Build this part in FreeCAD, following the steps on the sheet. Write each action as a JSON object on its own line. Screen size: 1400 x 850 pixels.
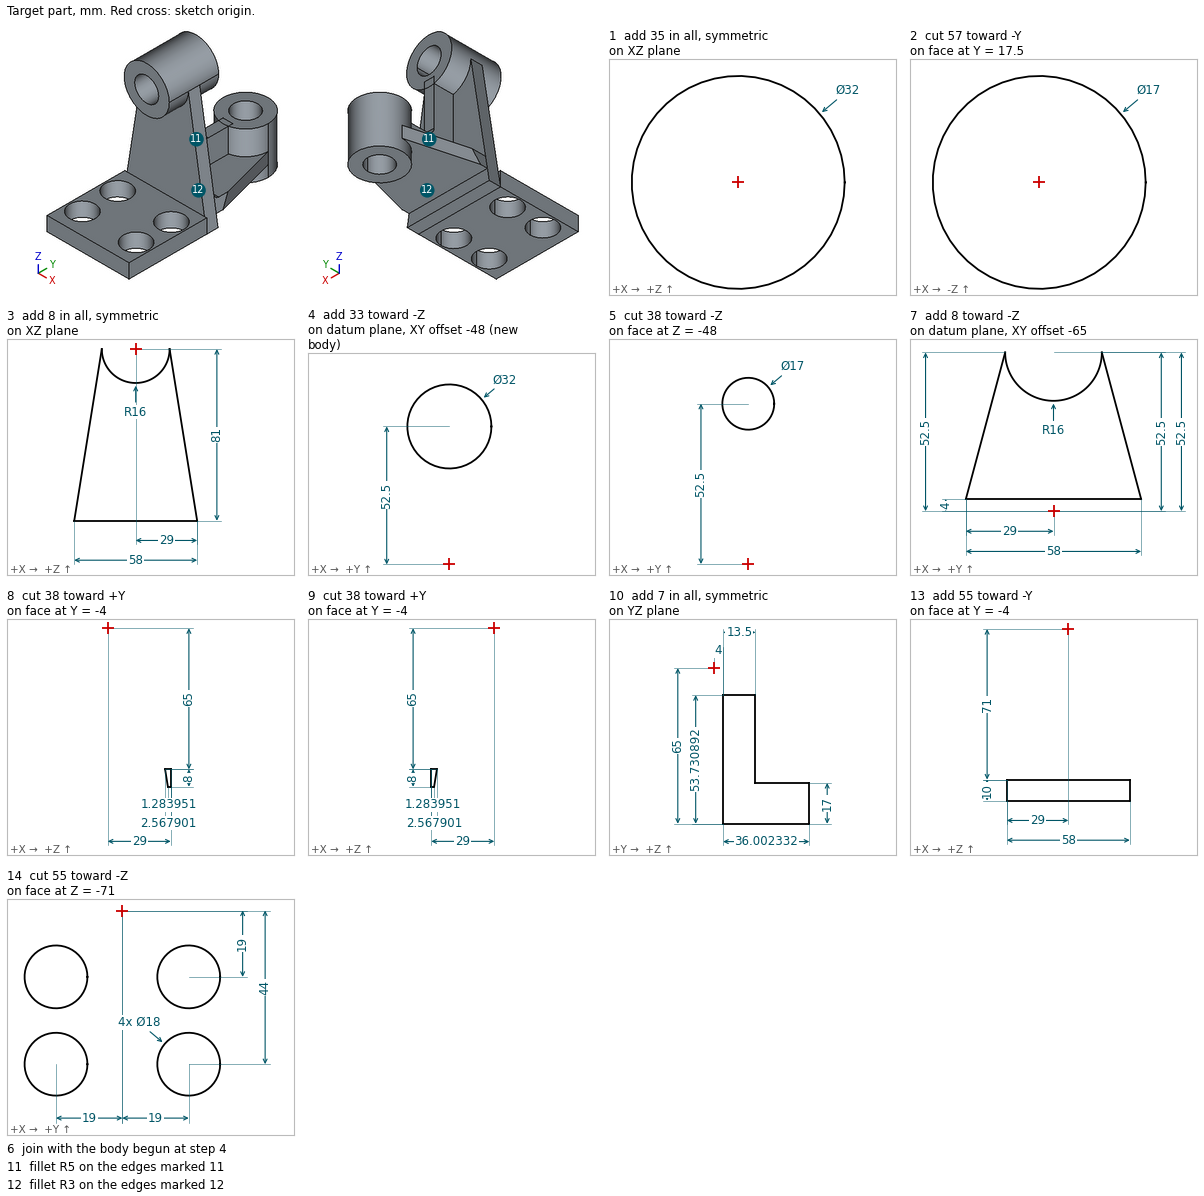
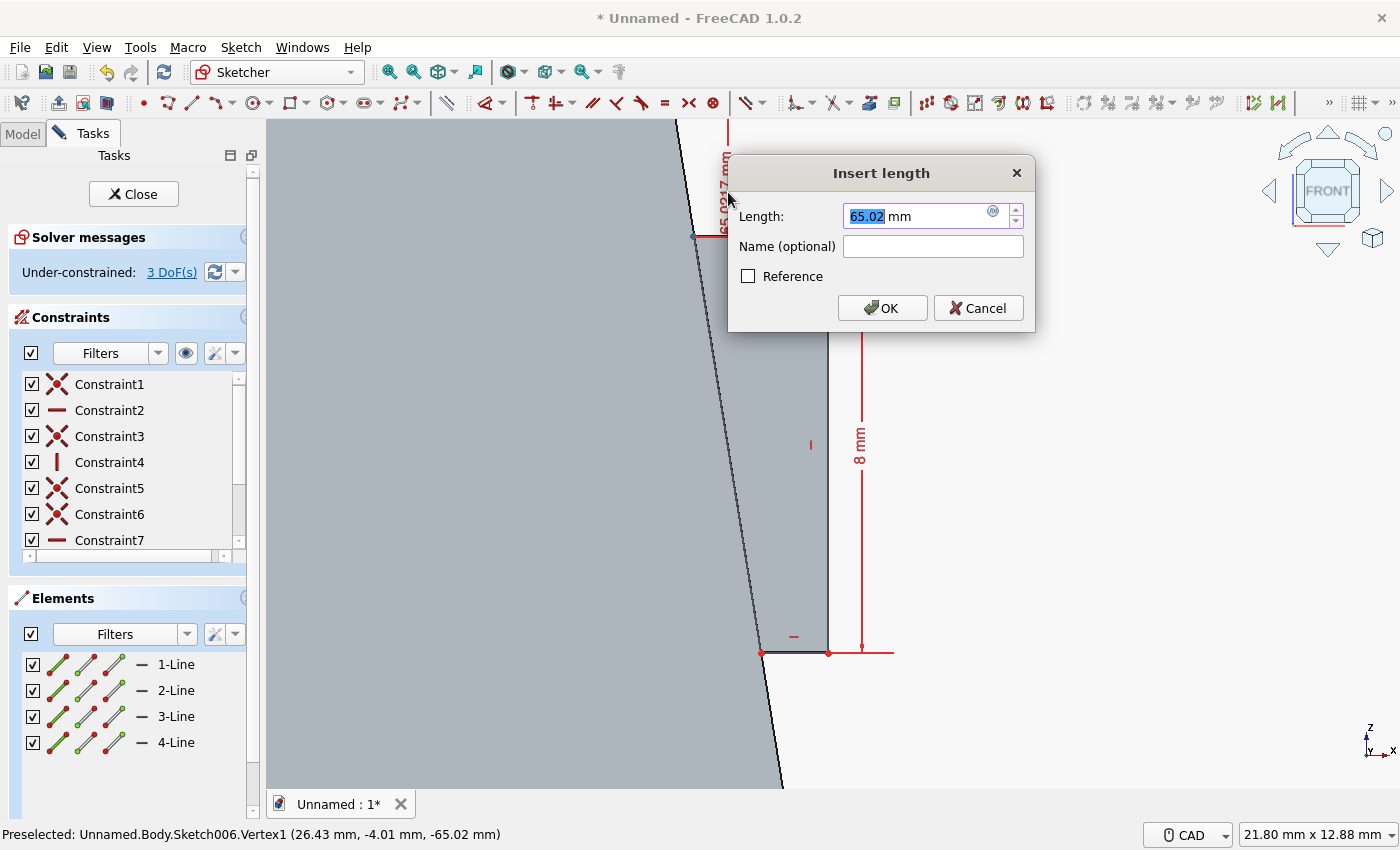
{"action": "type", "text": "65"}
{"action": "key", "text": "Return"}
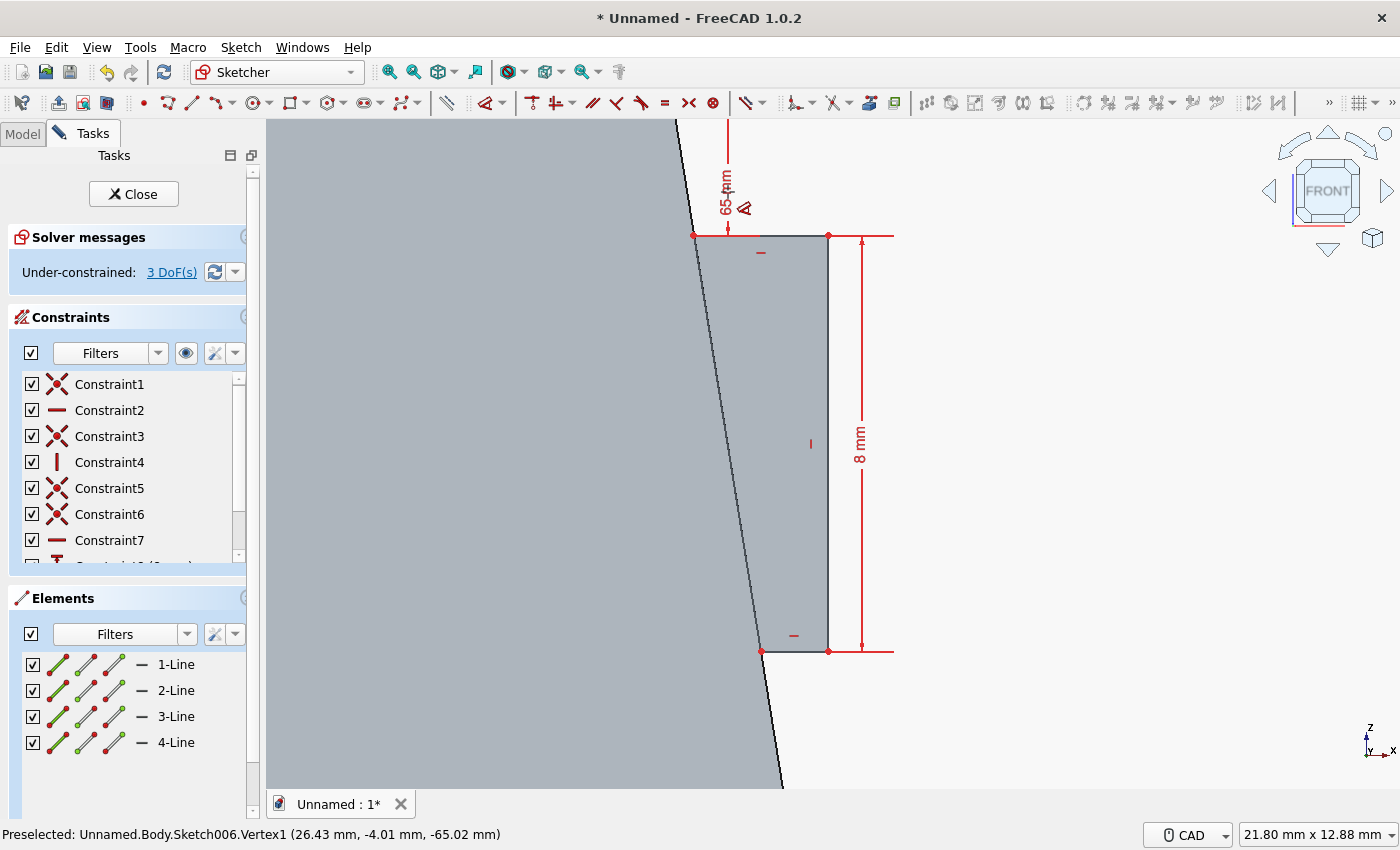
{"action": "left_click", "coordinate": [828, 652]}
{"action": "left_click", "coordinate": [561, 686]}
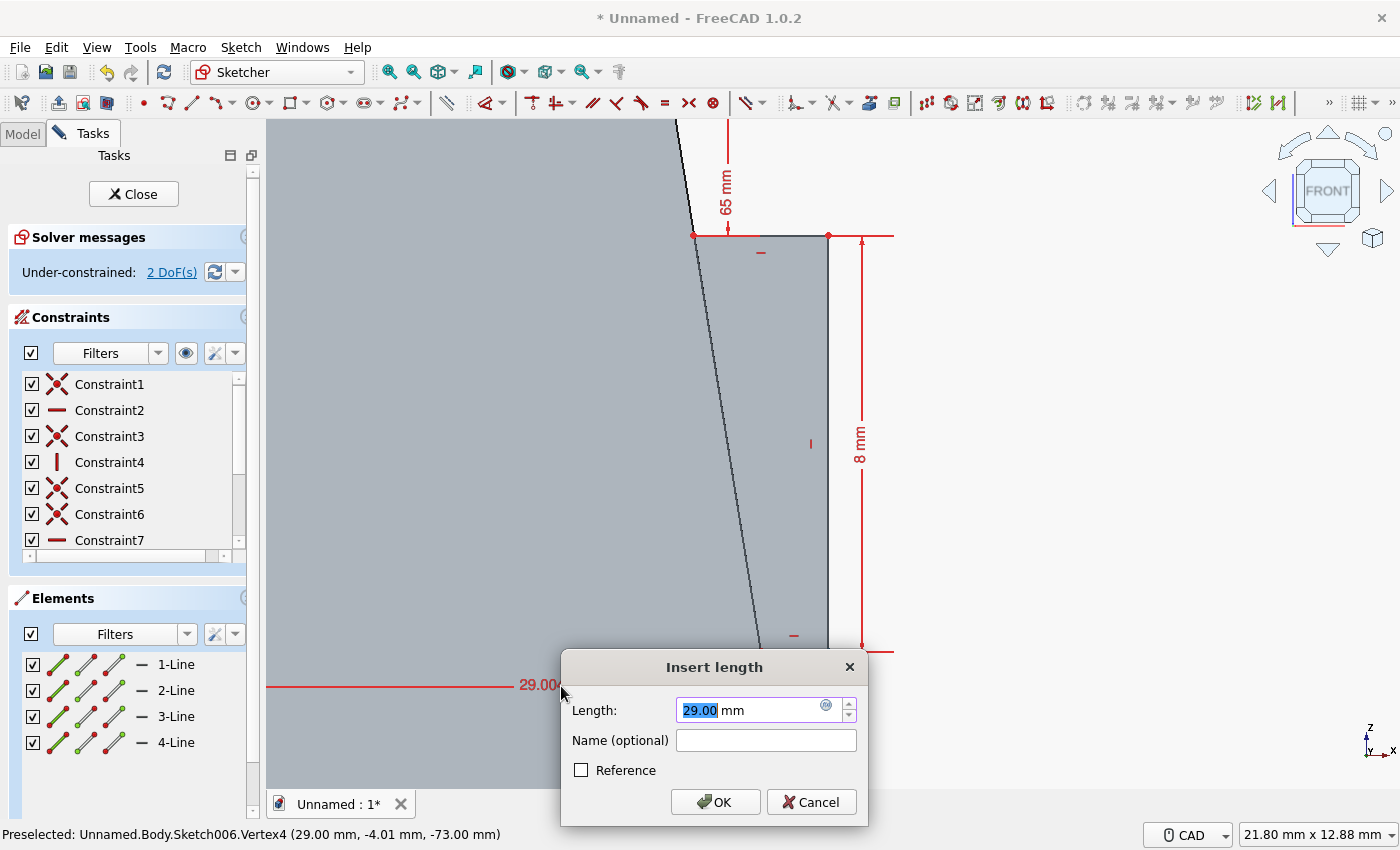
{"action": "type", "text": "29"}
{"action": "key", "text": "Return"}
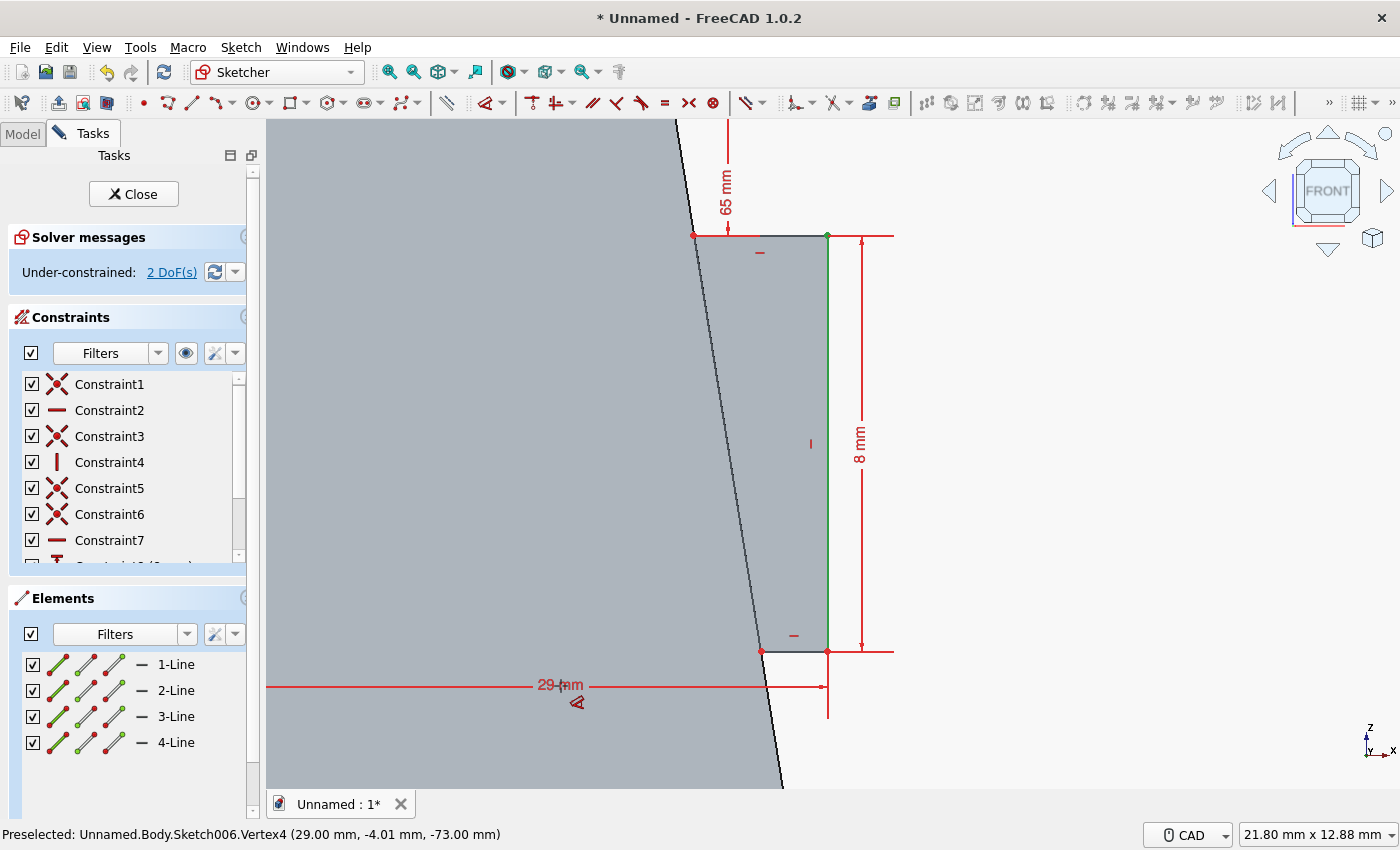
{"action": "left_click", "coordinate": [781, 652]}
{"action": "left_click", "coordinate": [794, 686]}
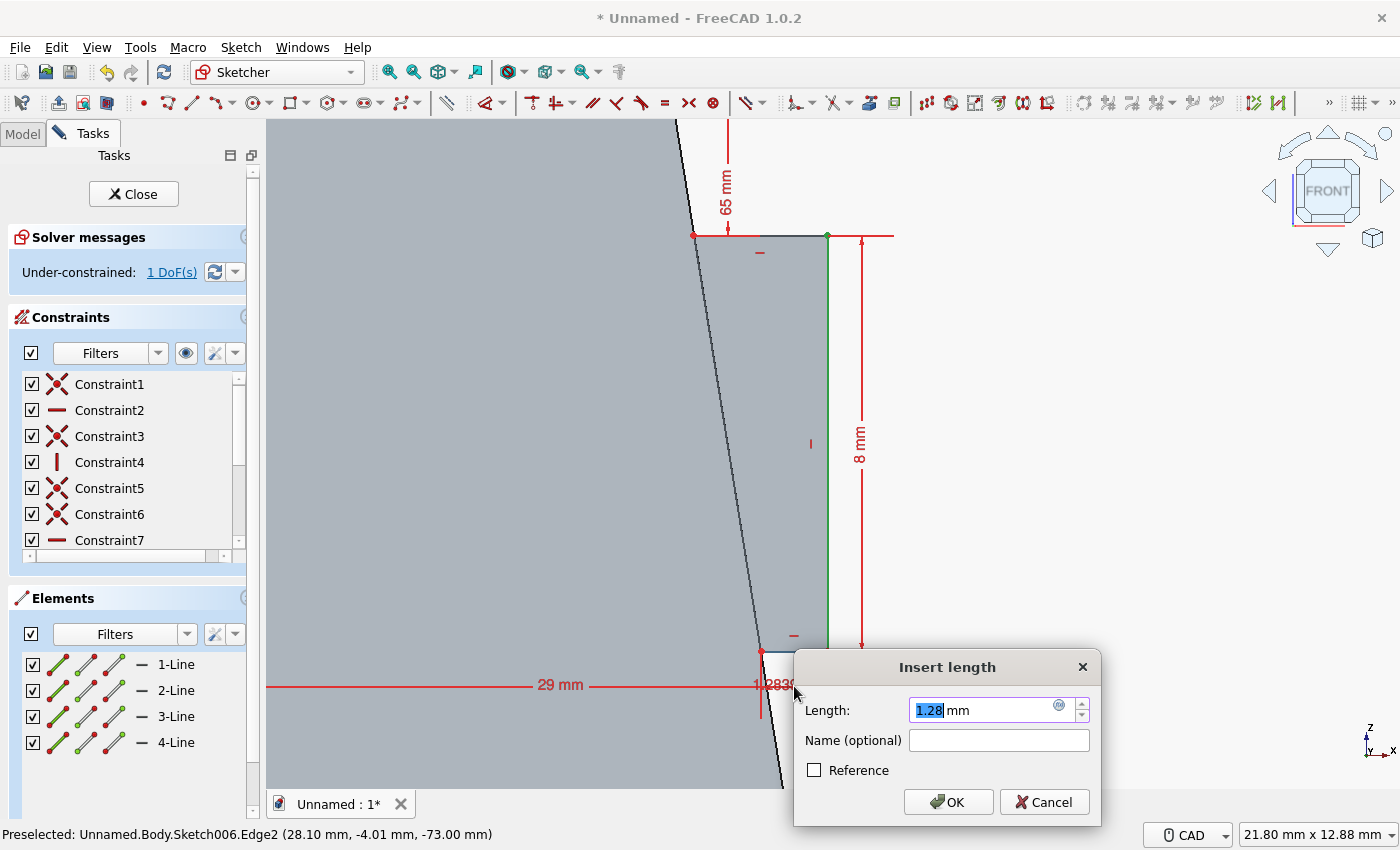
{"action": "type", "text": "1.283951"}
{"action": "key", "text": "Return"}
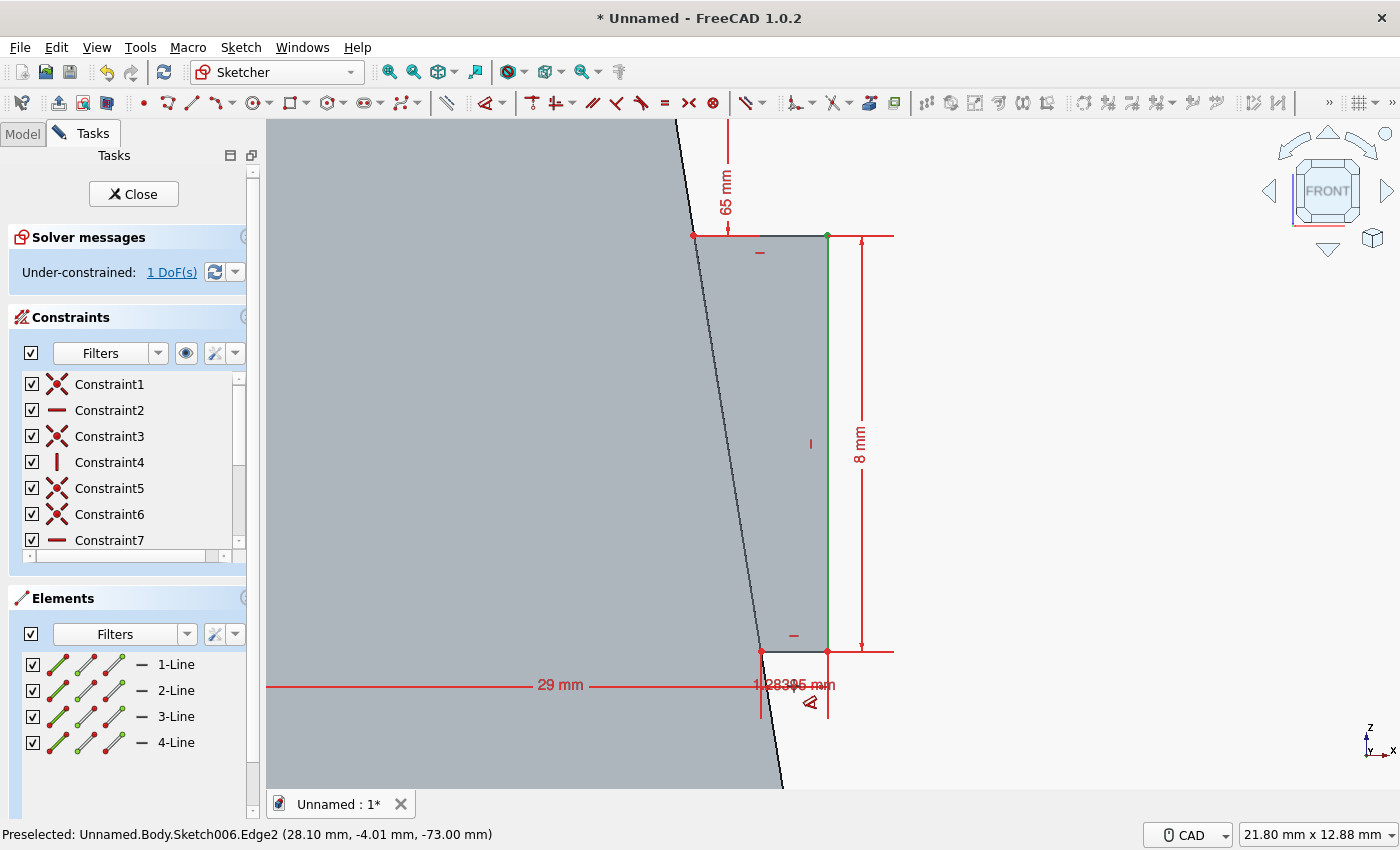
{"action": "left_click", "coordinate": [788, 236]}
{"action": "left_click", "coordinate": [808, 202]}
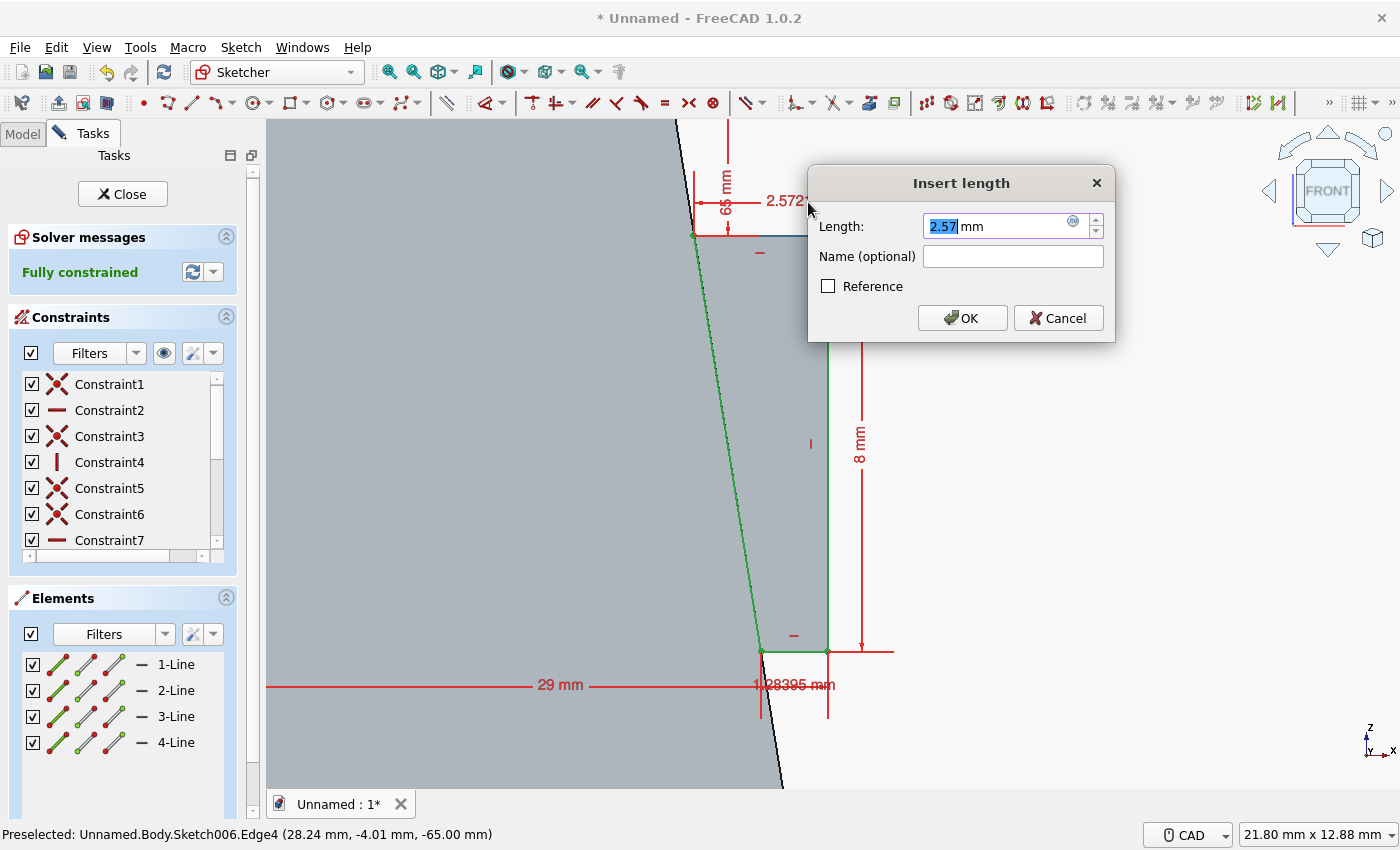
{"action": "type", "text": "2.567901"}
{"action": "key", "text": "Return"}
{"action": "key", "text": "Escape"}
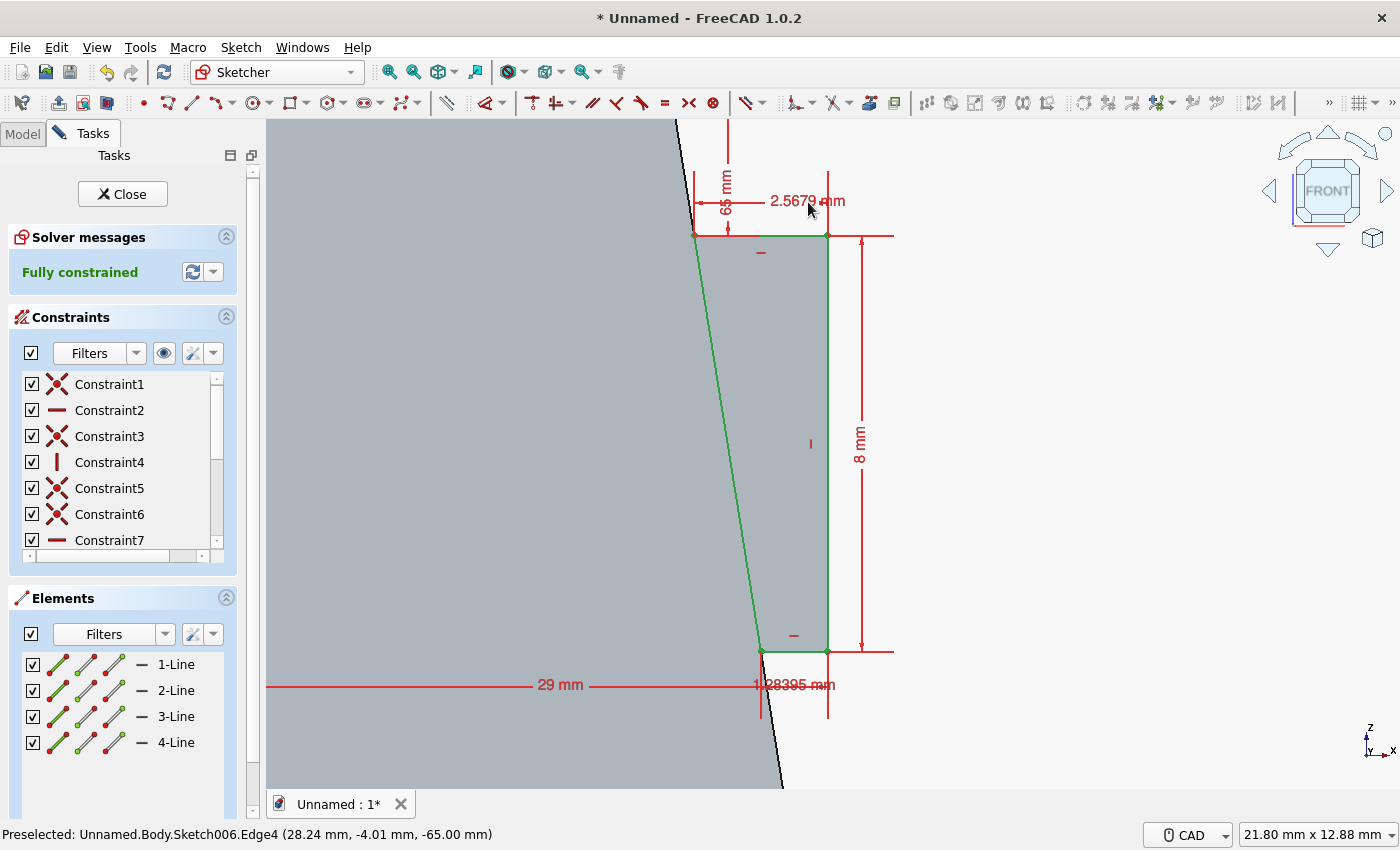
{"action": "left_click", "coordinate": [123, 194]}